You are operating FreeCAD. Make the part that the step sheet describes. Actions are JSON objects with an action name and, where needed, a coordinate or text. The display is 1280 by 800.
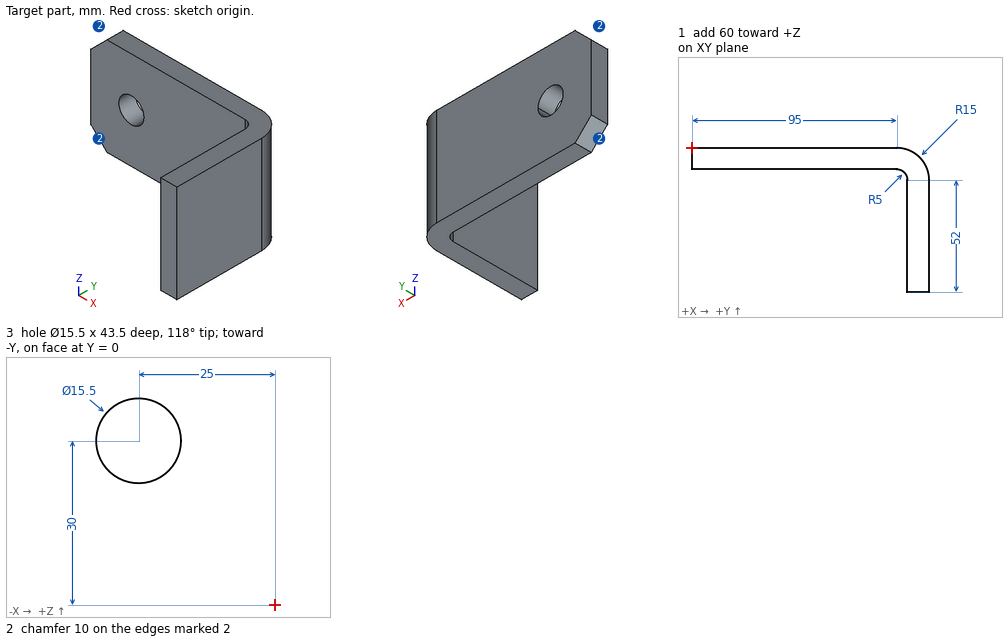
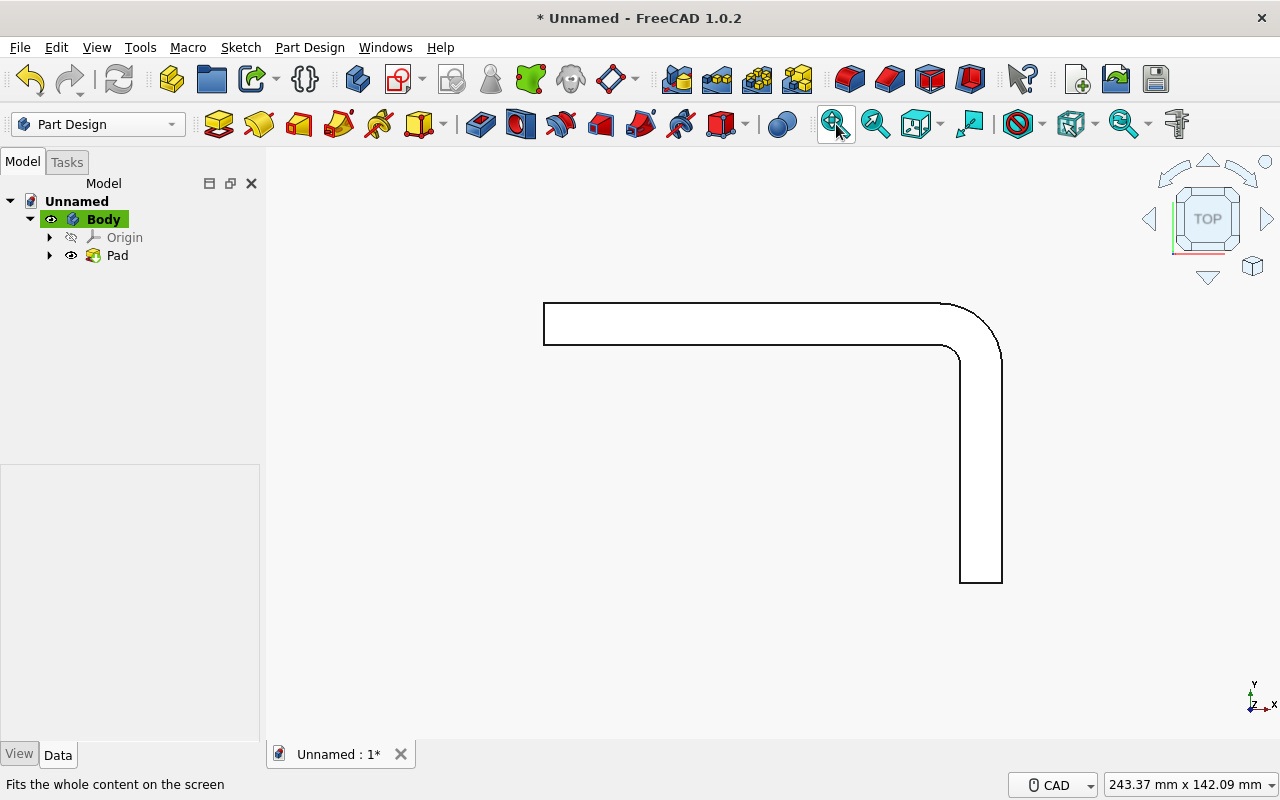
{"action": "left_click", "coordinate": [544, 323]}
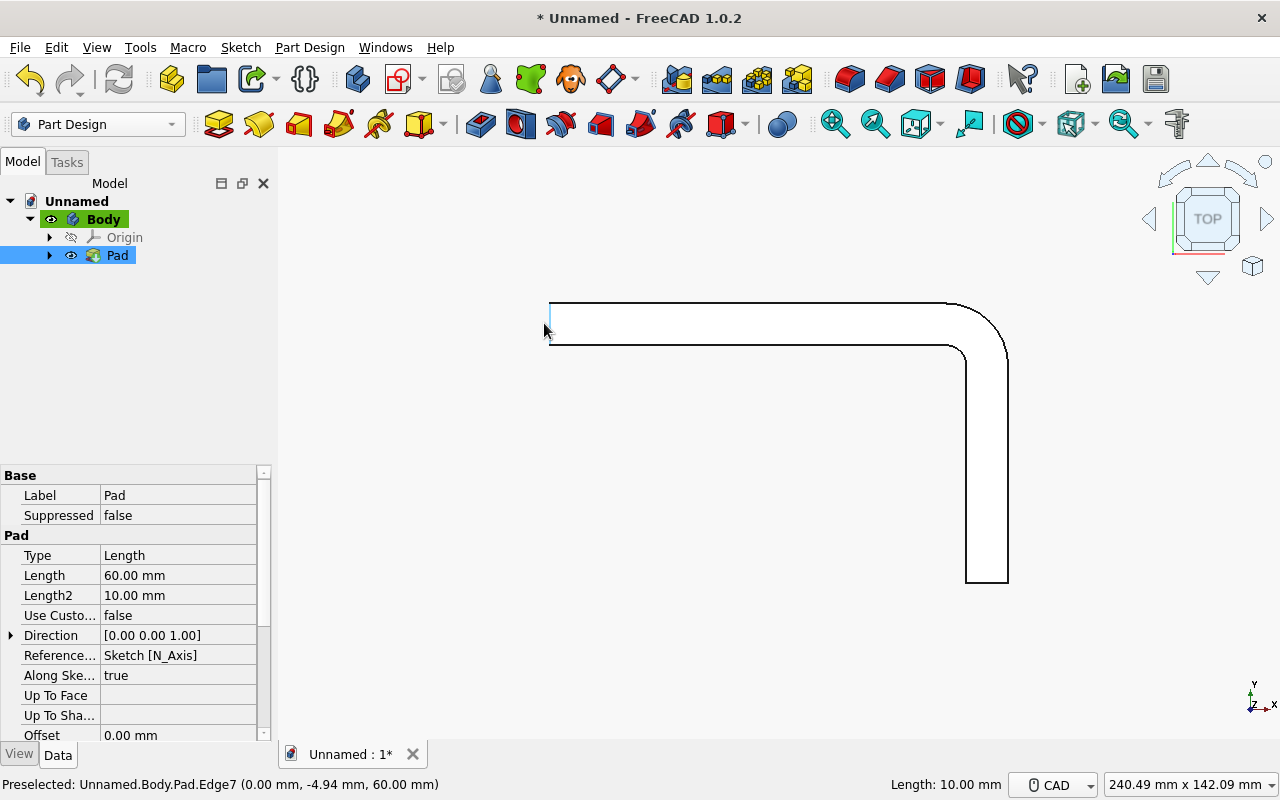
{"action": "key", "text": "1"}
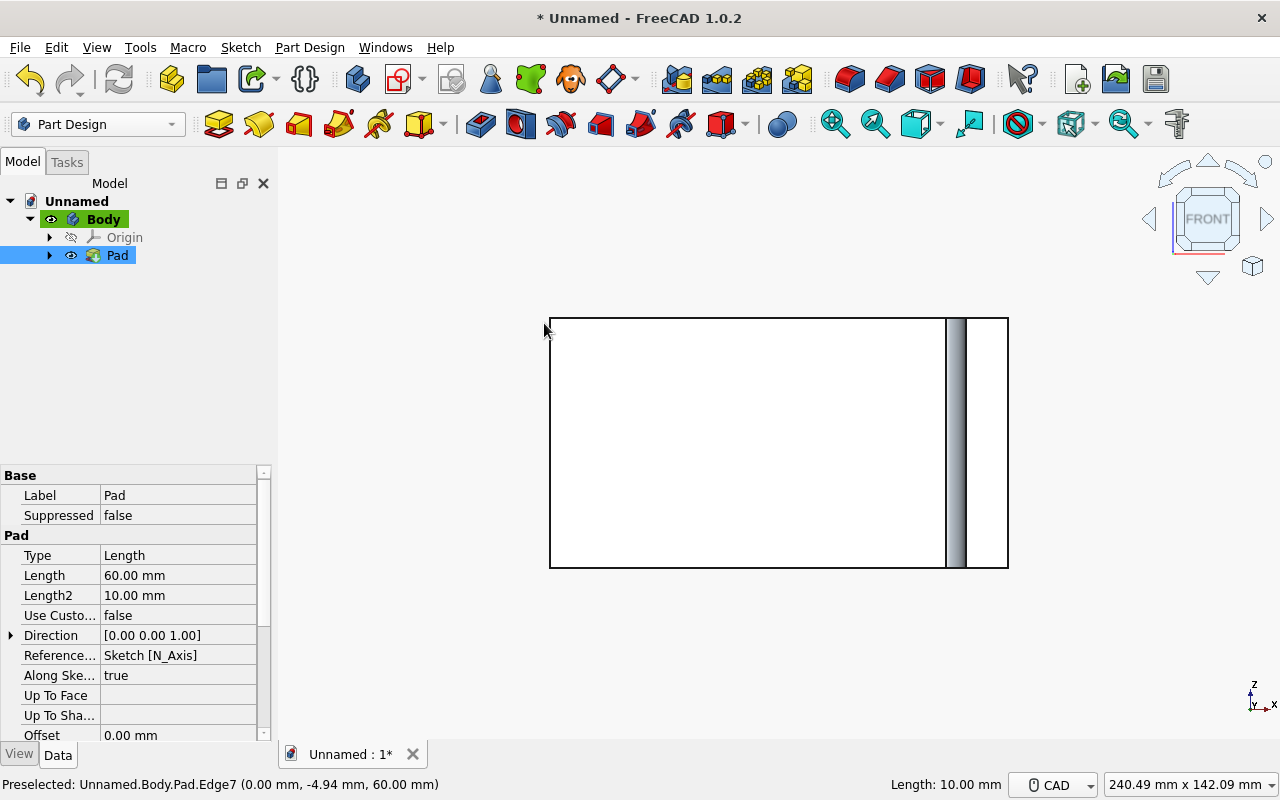
{"action": "key", "text": "3"}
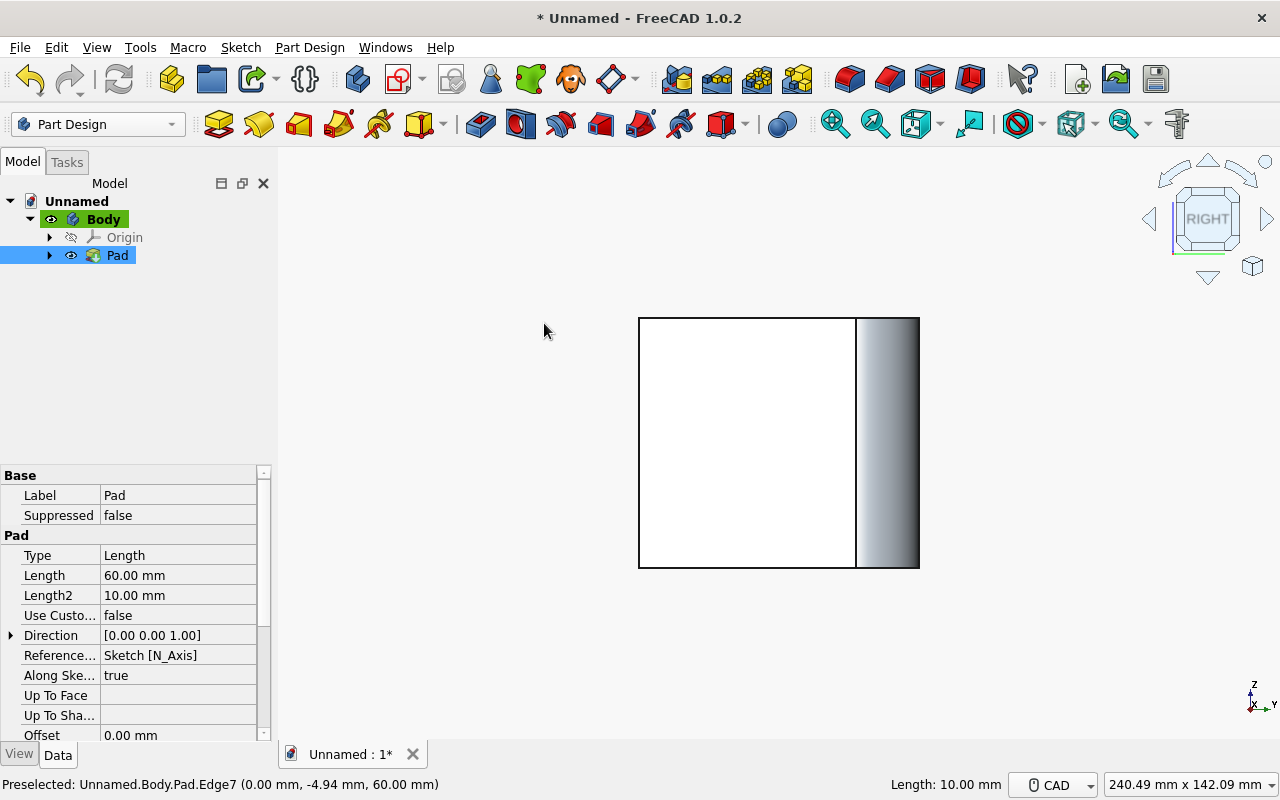
{"action": "left_click", "coordinate": [836, 124]}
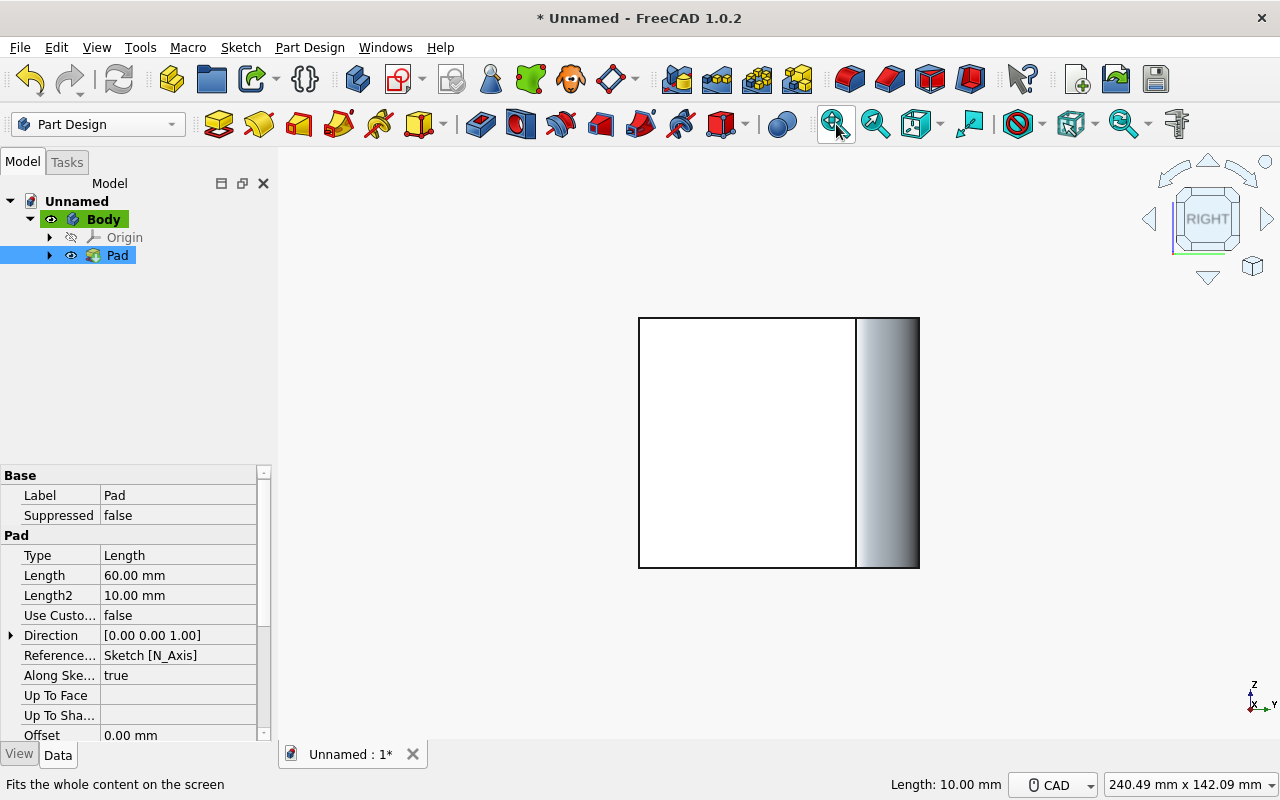
{"action": "key", "text": "5"}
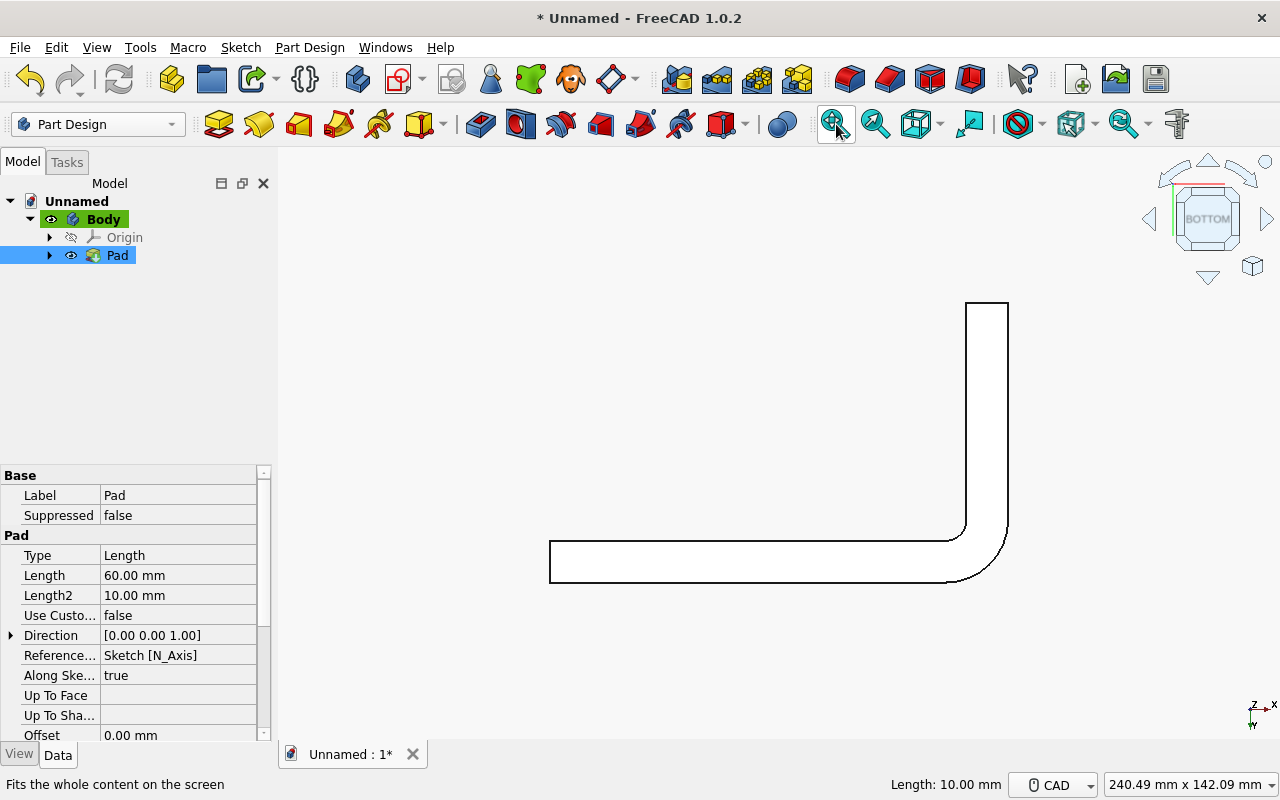
{"action": "left_click", "coordinate": [550, 561], "text": "ctrl"}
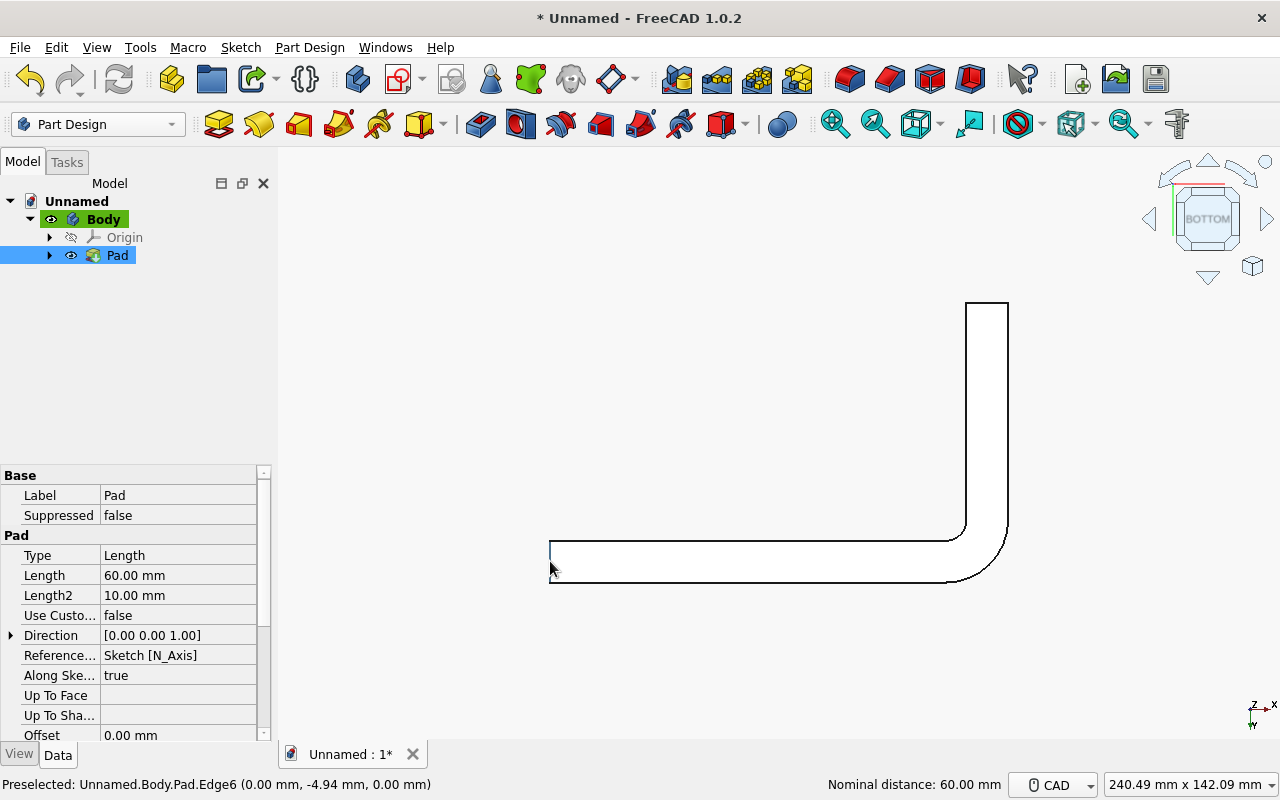
{"action": "left_click", "coordinate": [890, 80]}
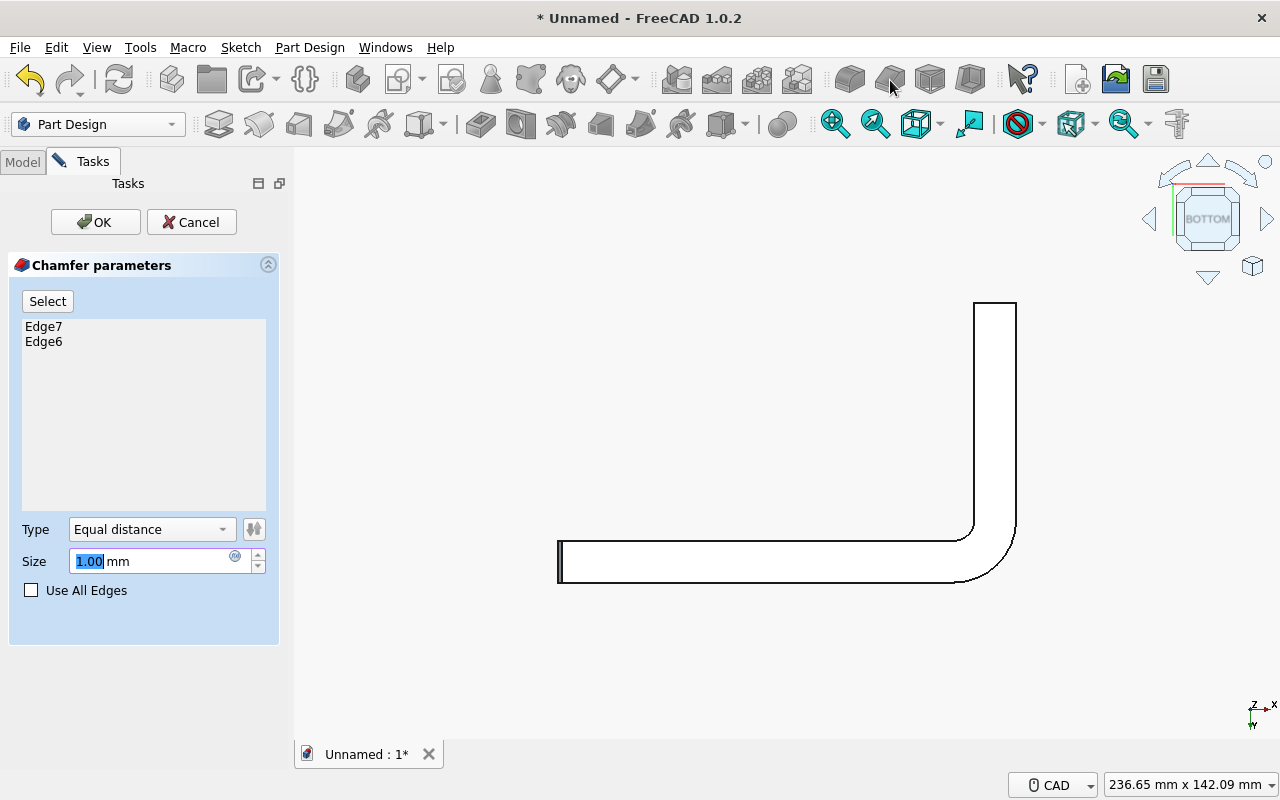
{"action": "type", "text": "10"}
{"action": "key", "text": "Tab"}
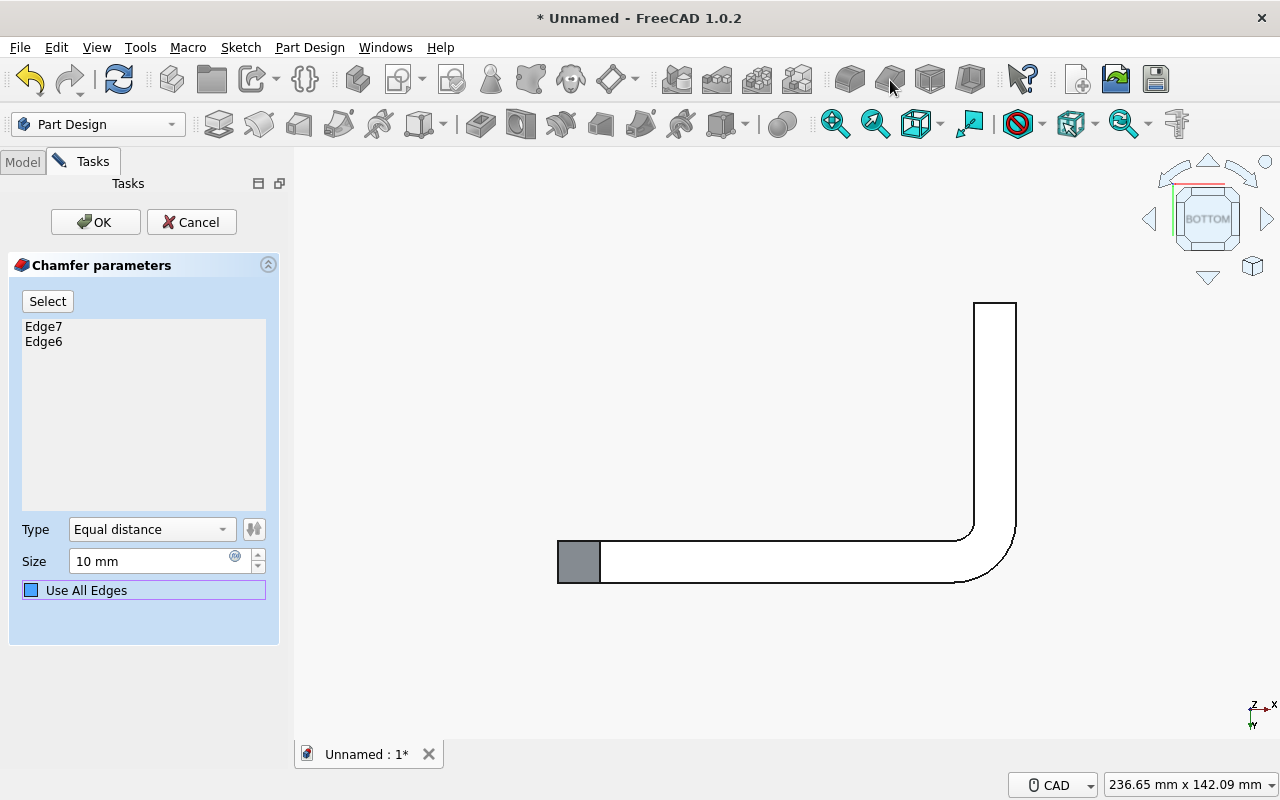
{"action": "left_click", "coordinate": [96, 222]}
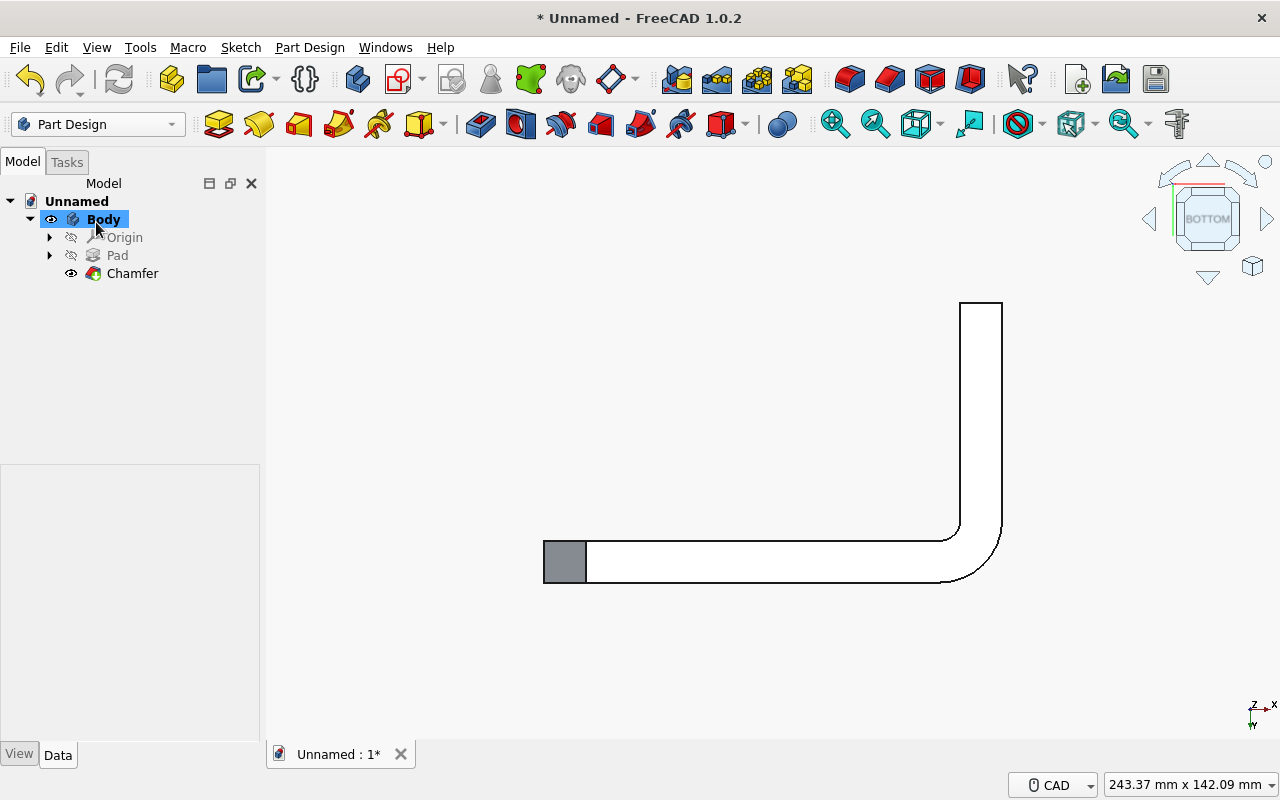
{"action": "key", "text": "4"}